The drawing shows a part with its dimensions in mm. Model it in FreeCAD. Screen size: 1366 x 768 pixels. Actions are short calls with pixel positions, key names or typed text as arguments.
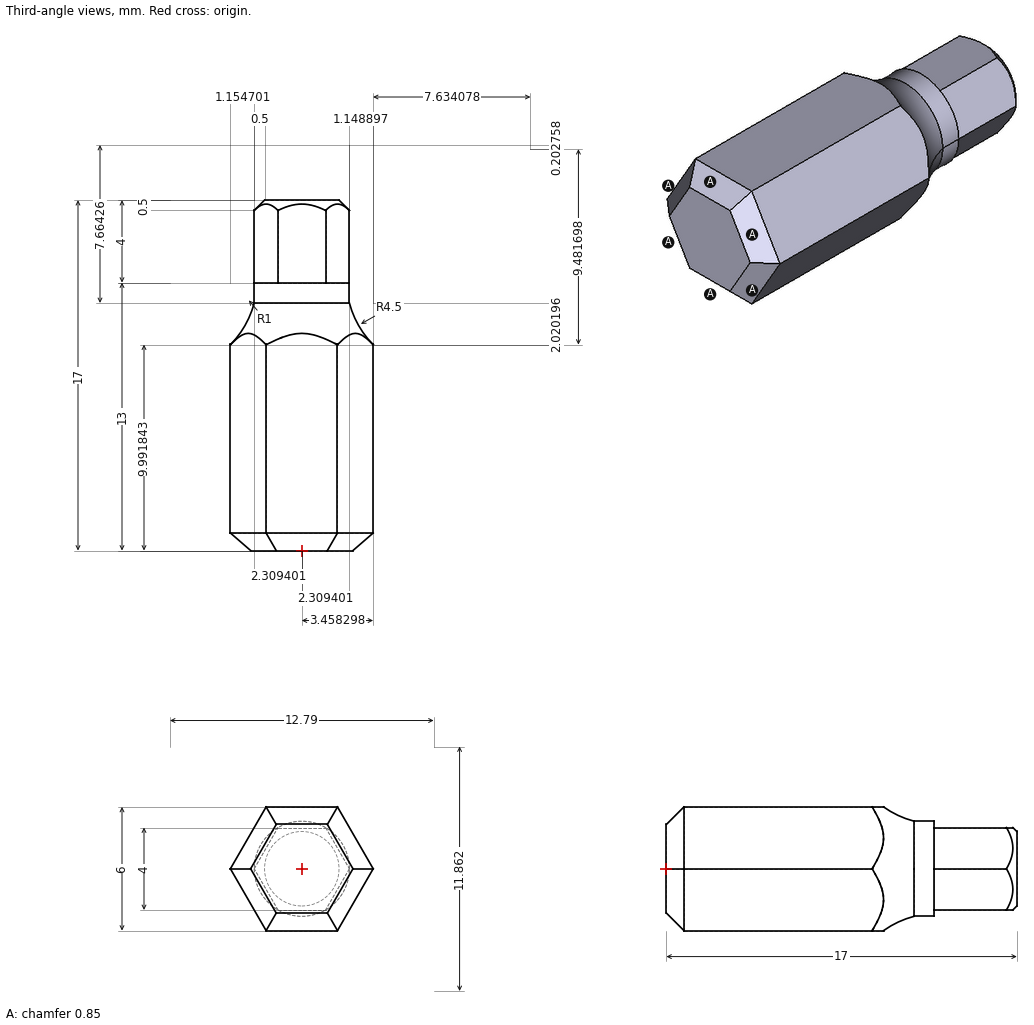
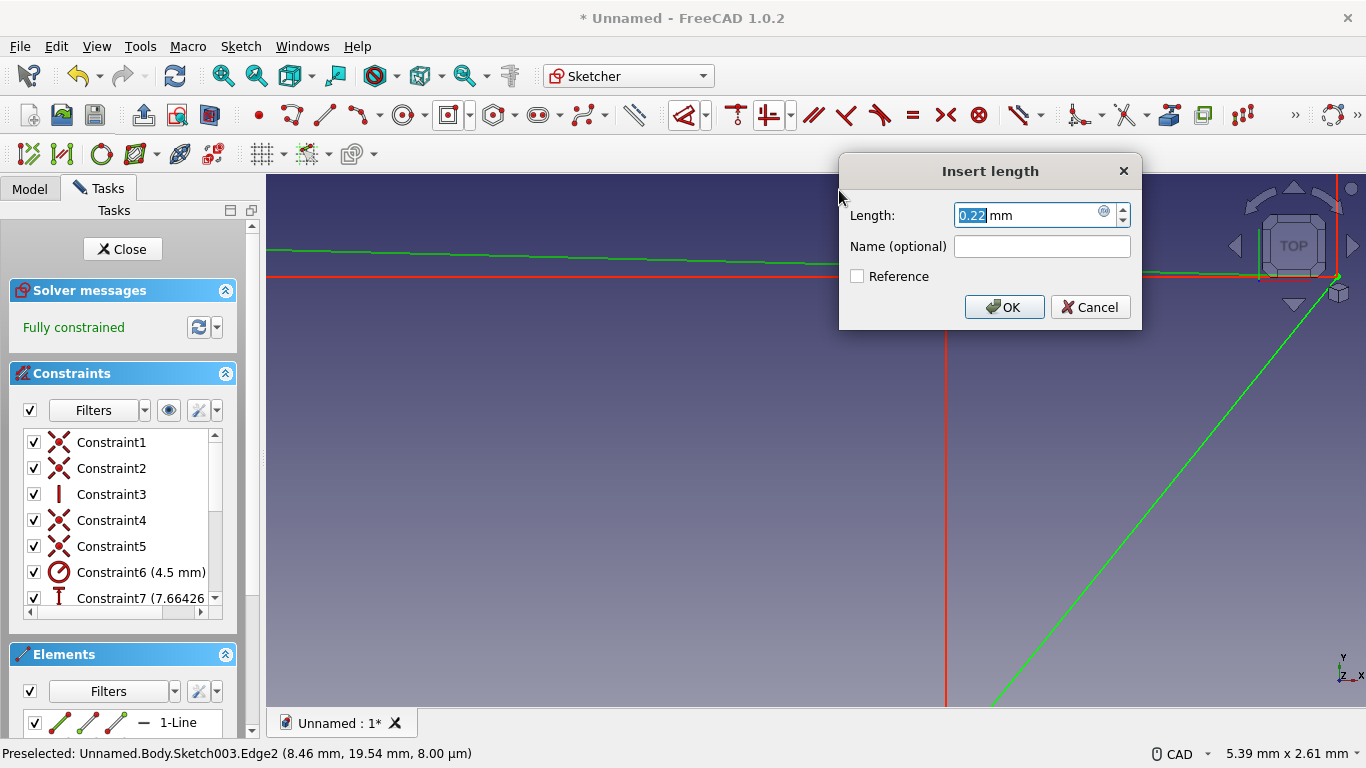
text(0.202758)
key(Return)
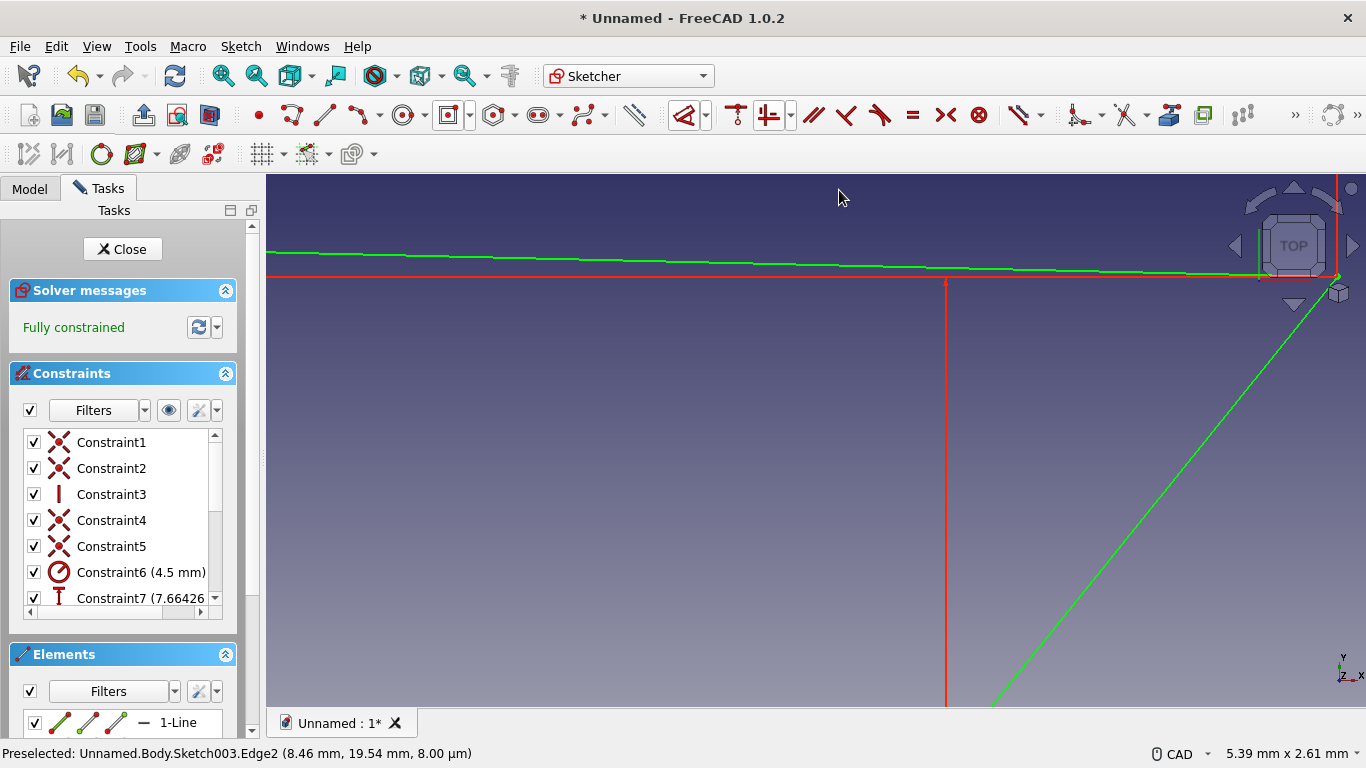
click(123, 249)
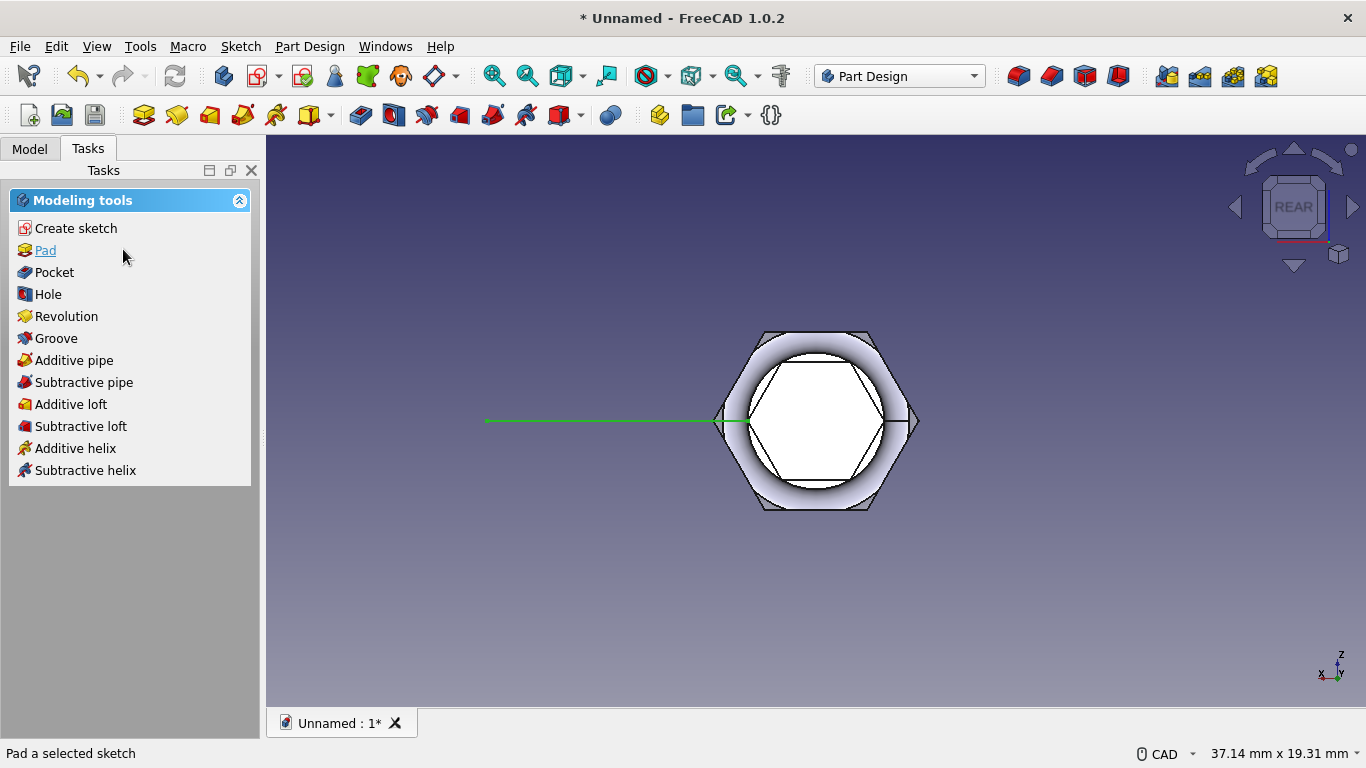
click(427, 116)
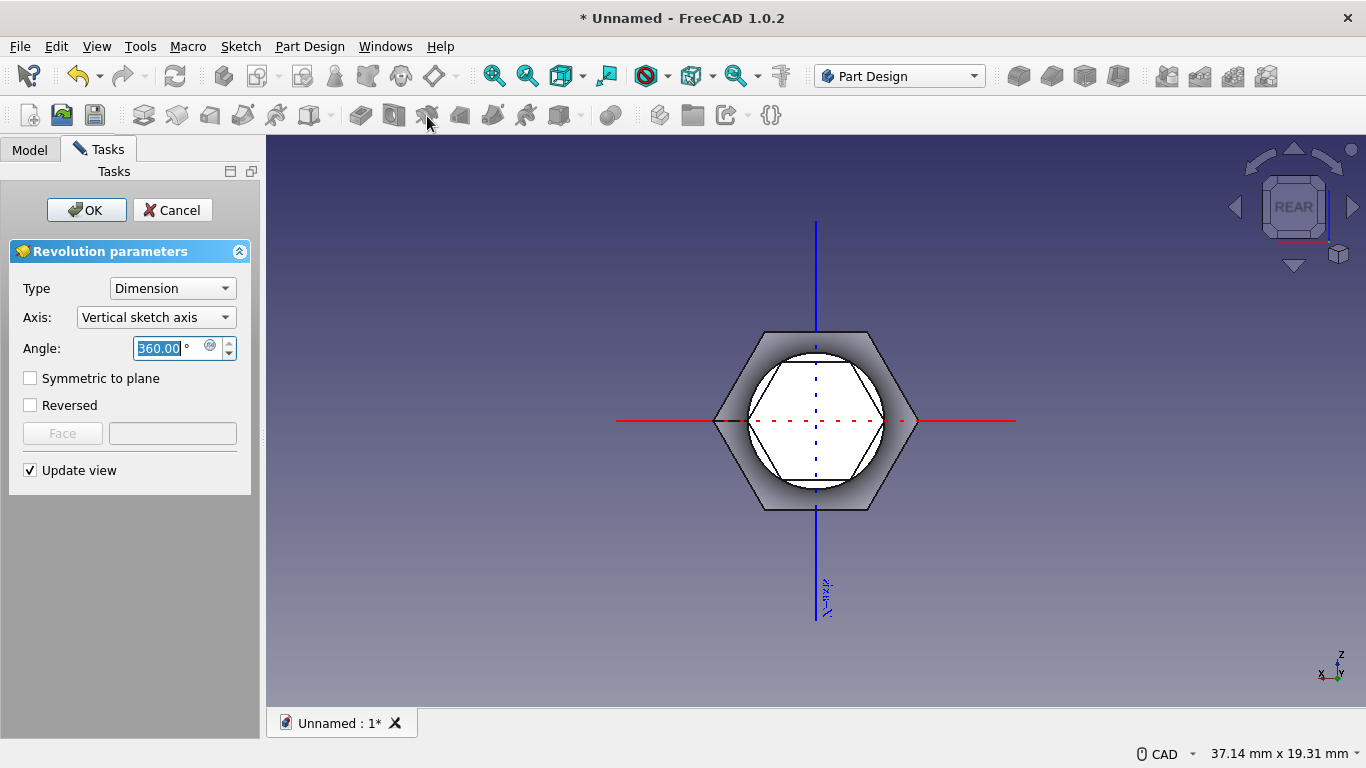
click(87, 210)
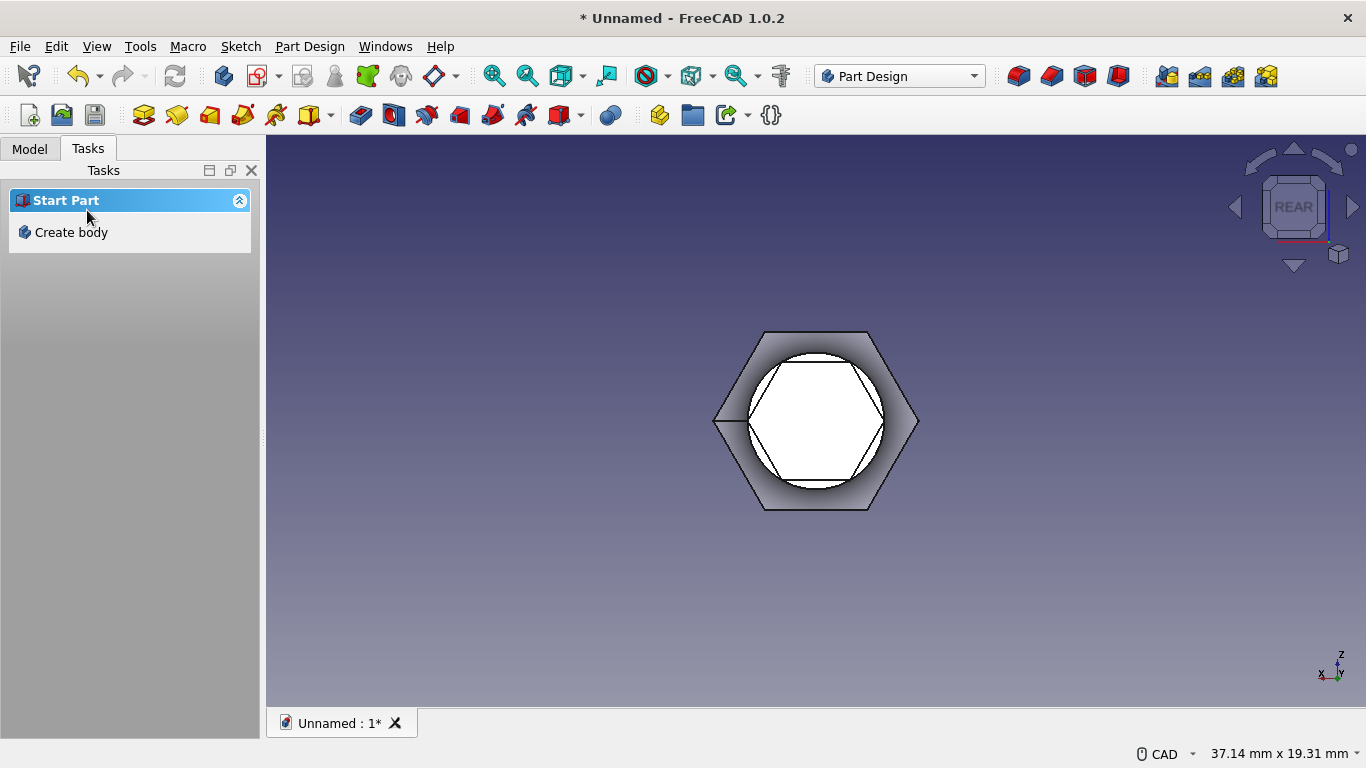
click(495, 76)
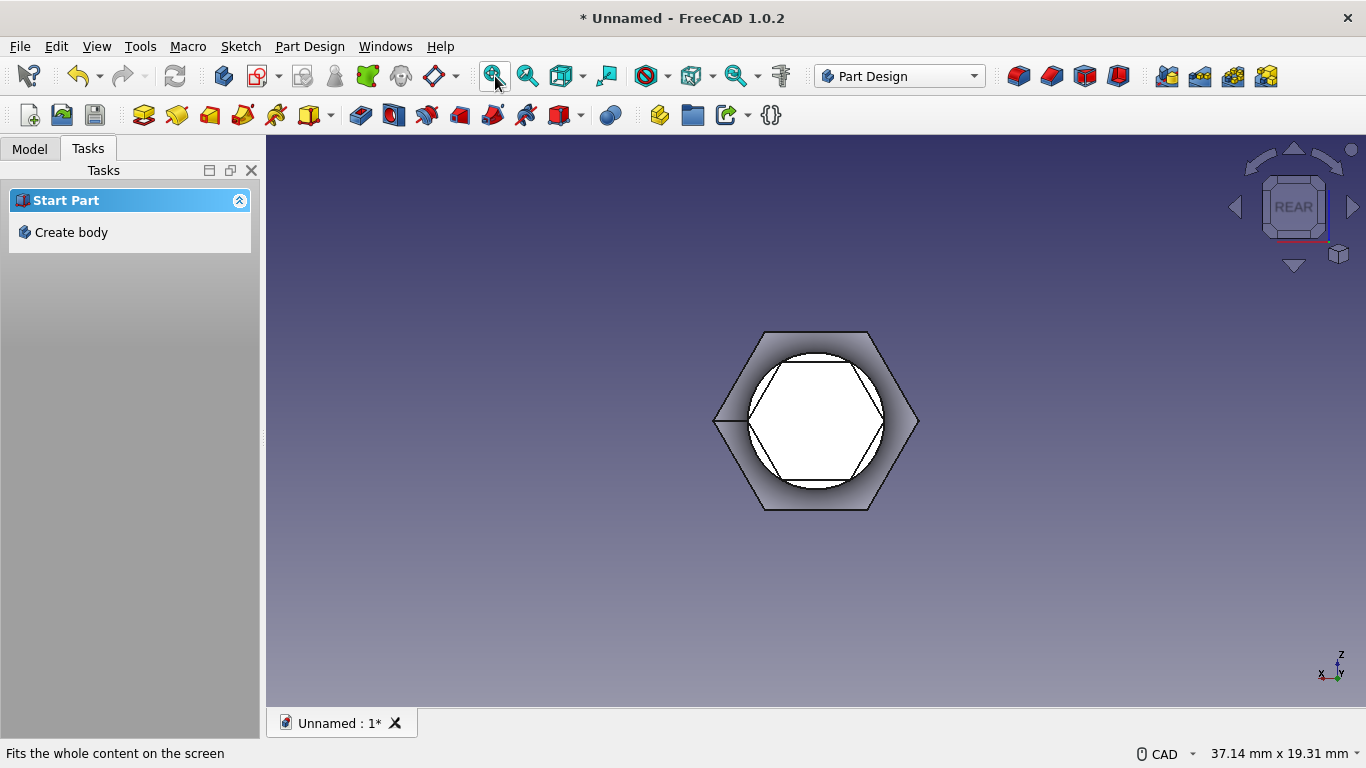
click(256, 76)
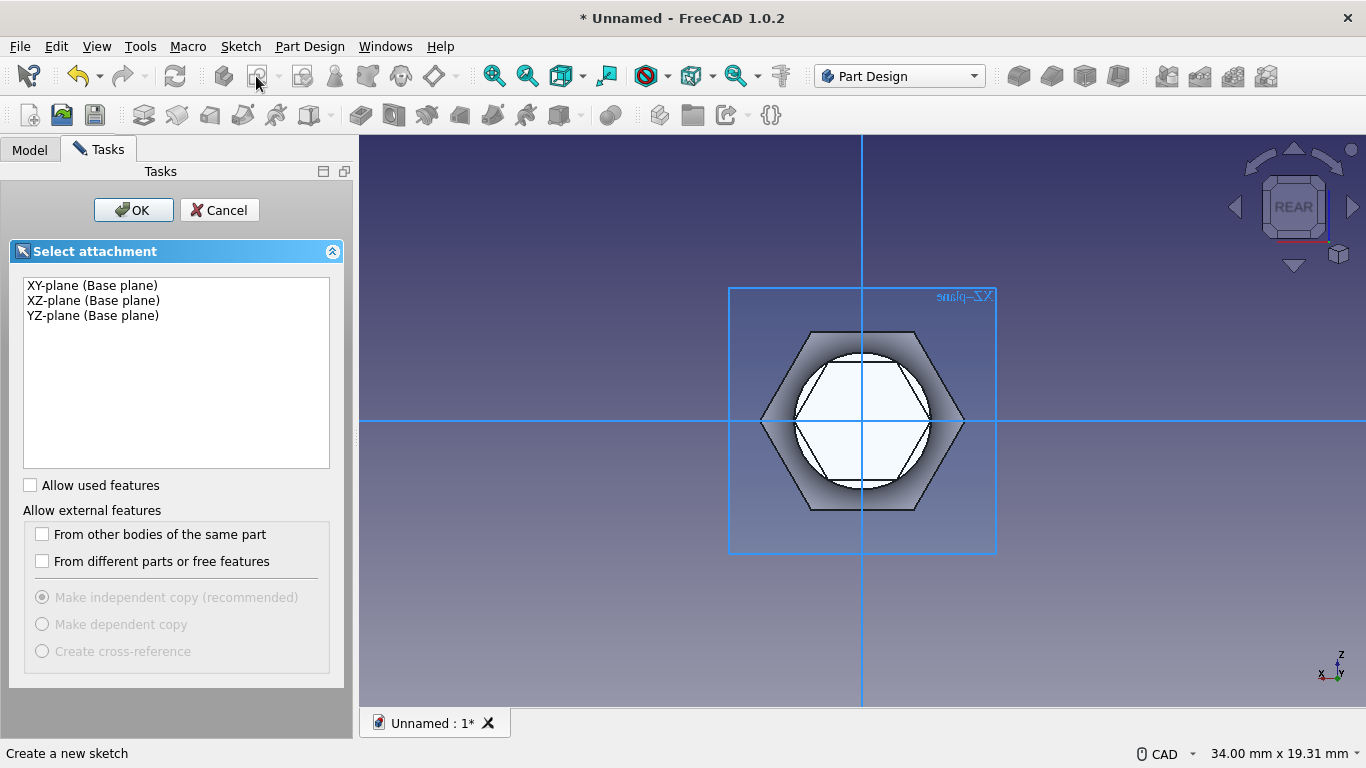
click(84, 286)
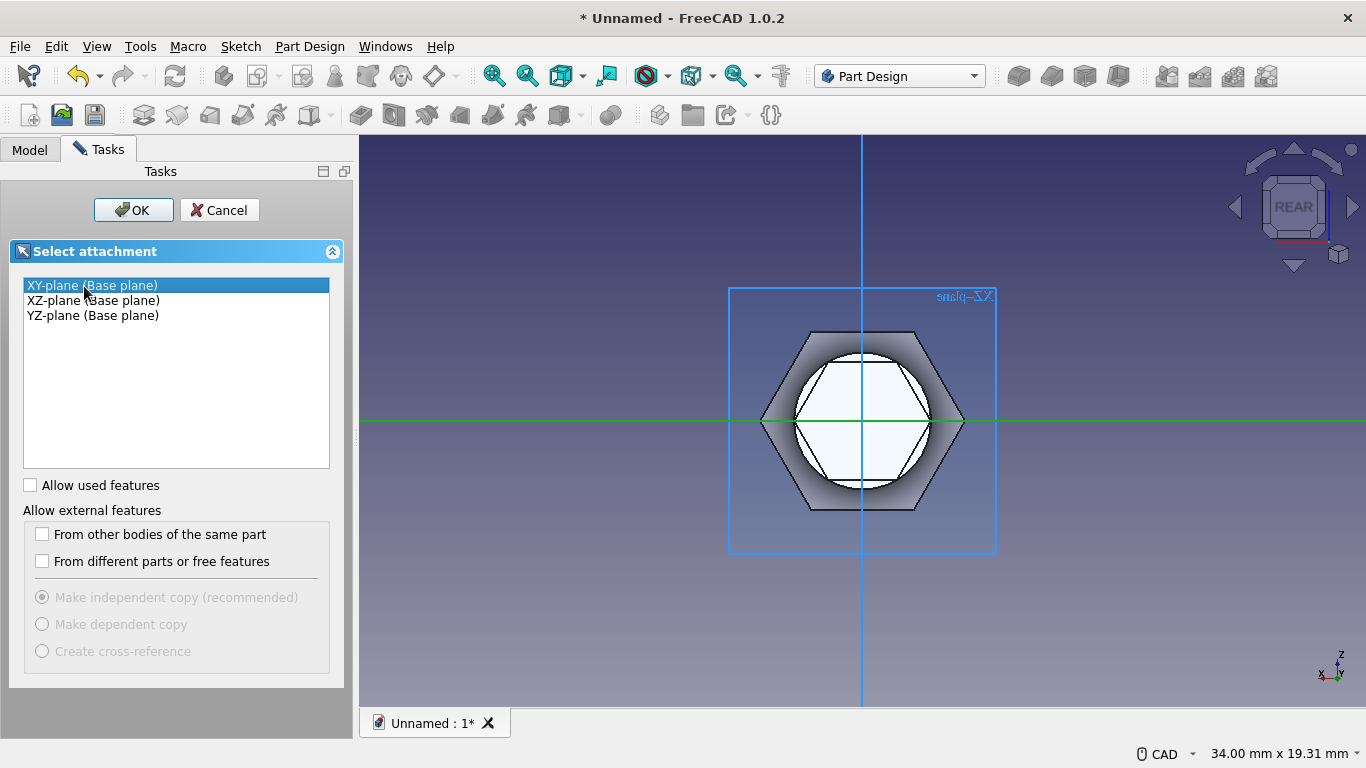
click(134, 210)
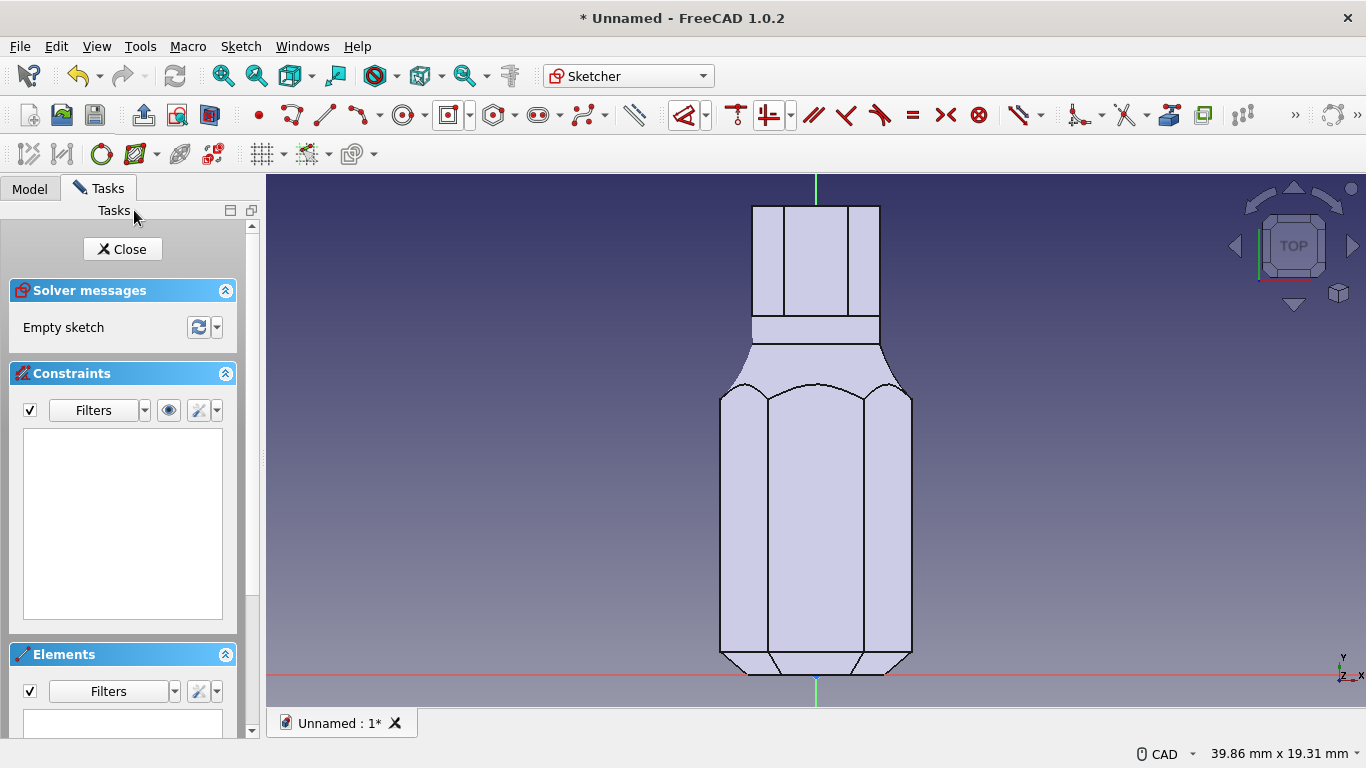
click(210, 116)